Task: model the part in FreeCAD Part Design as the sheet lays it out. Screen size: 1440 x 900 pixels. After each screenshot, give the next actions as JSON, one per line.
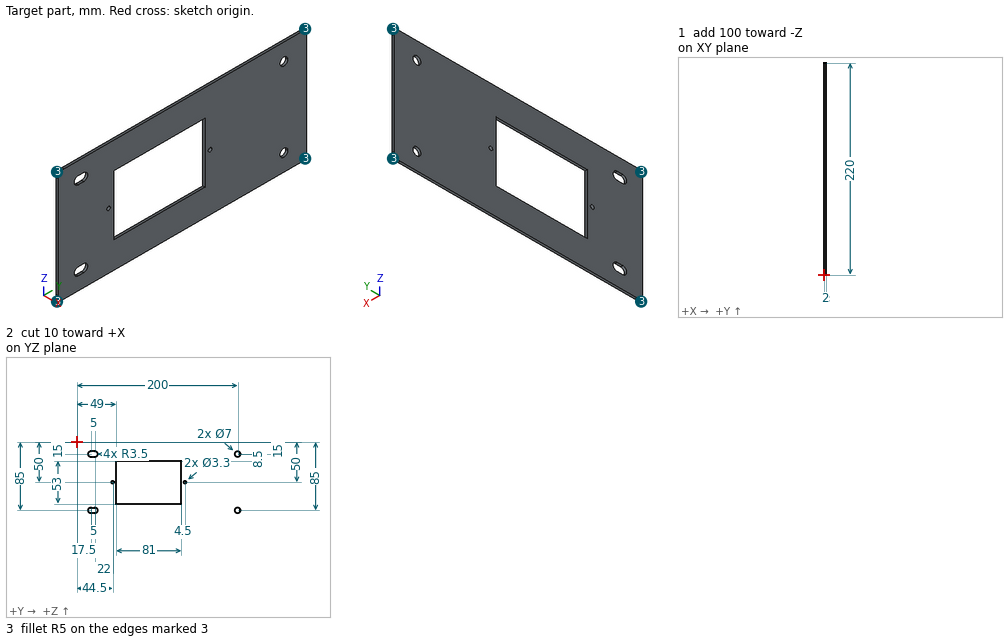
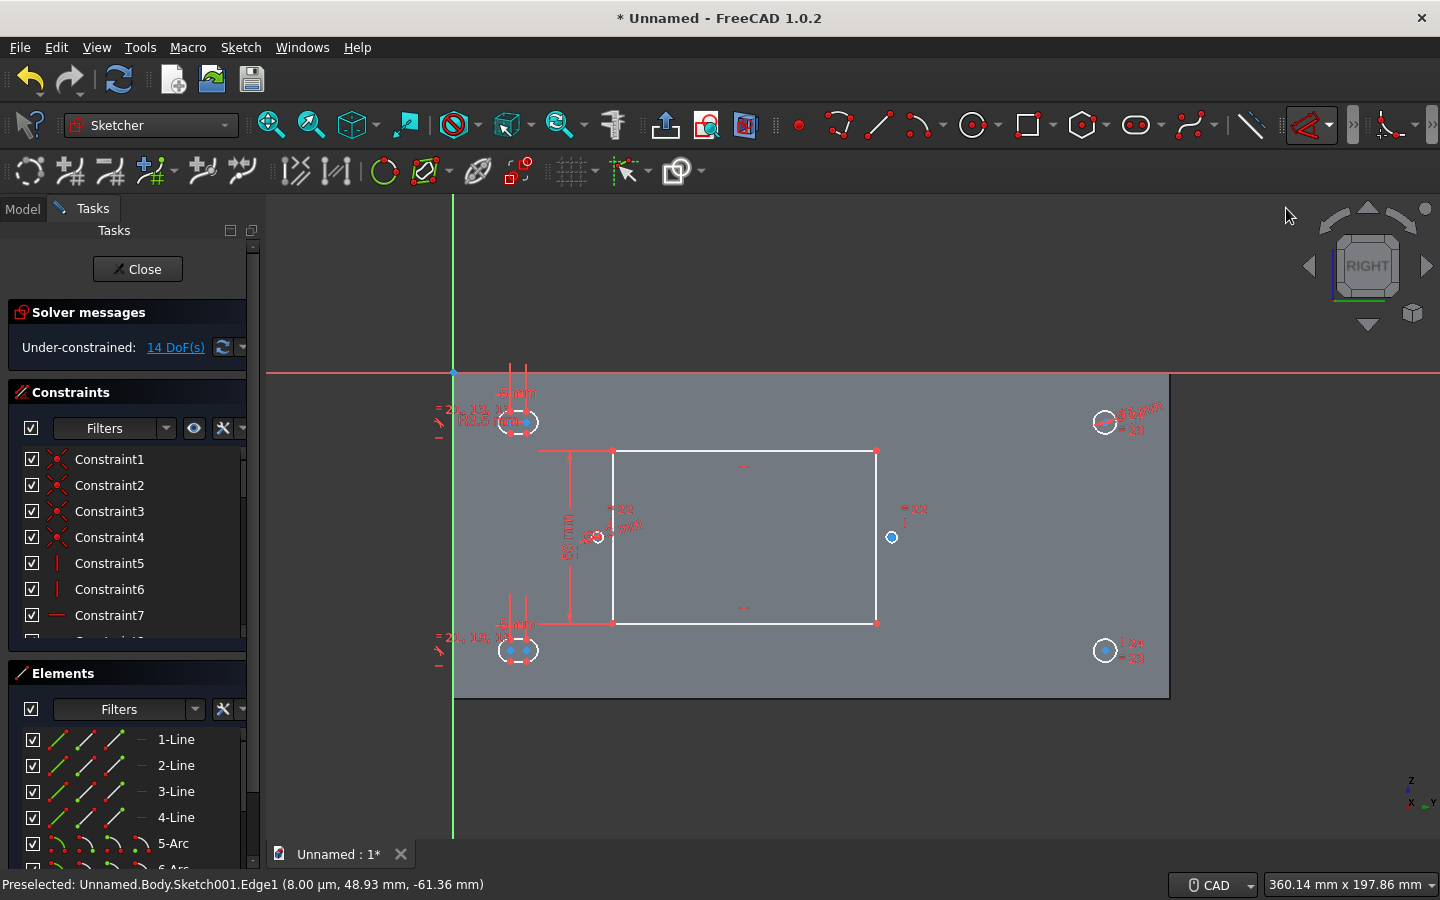
{"action": "left_click", "coordinate": [692, 624]}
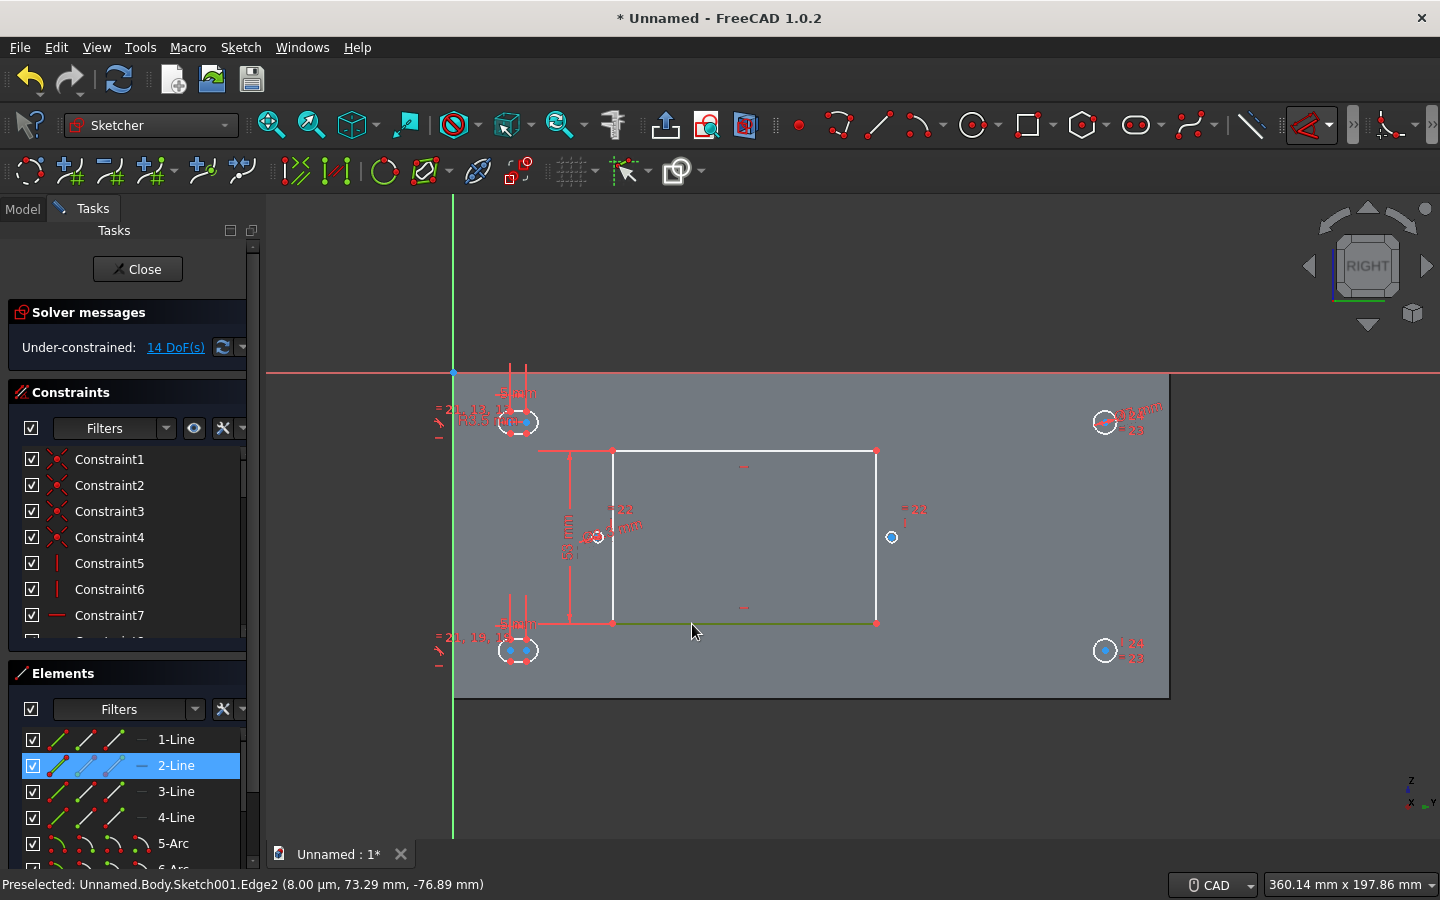
{"action": "left_click", "coordinate": [1332, 126]}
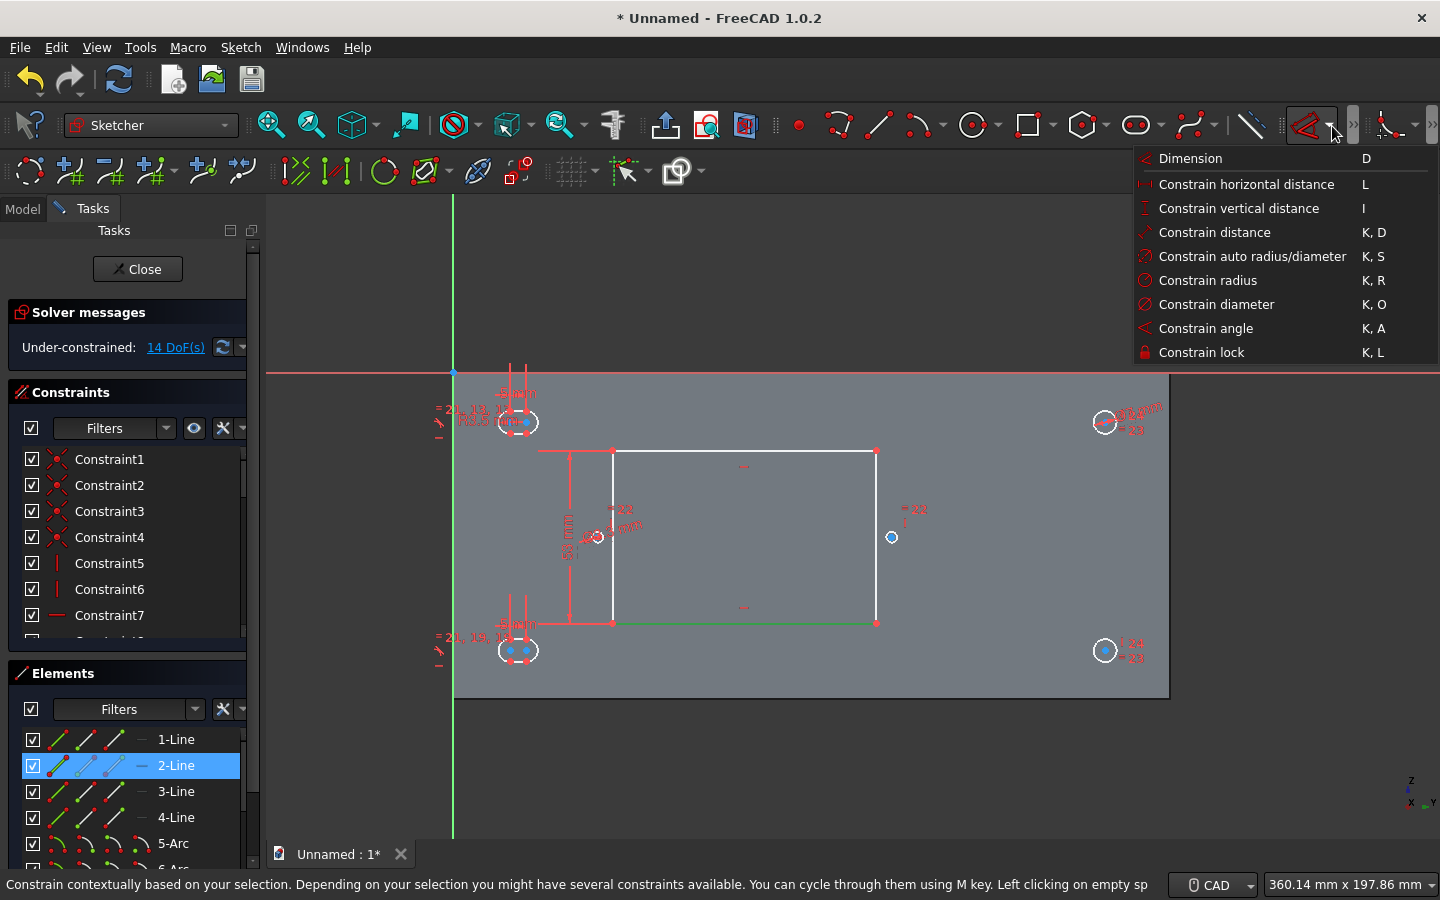
{"action": "left_click", "coordinate": [1286, 184]}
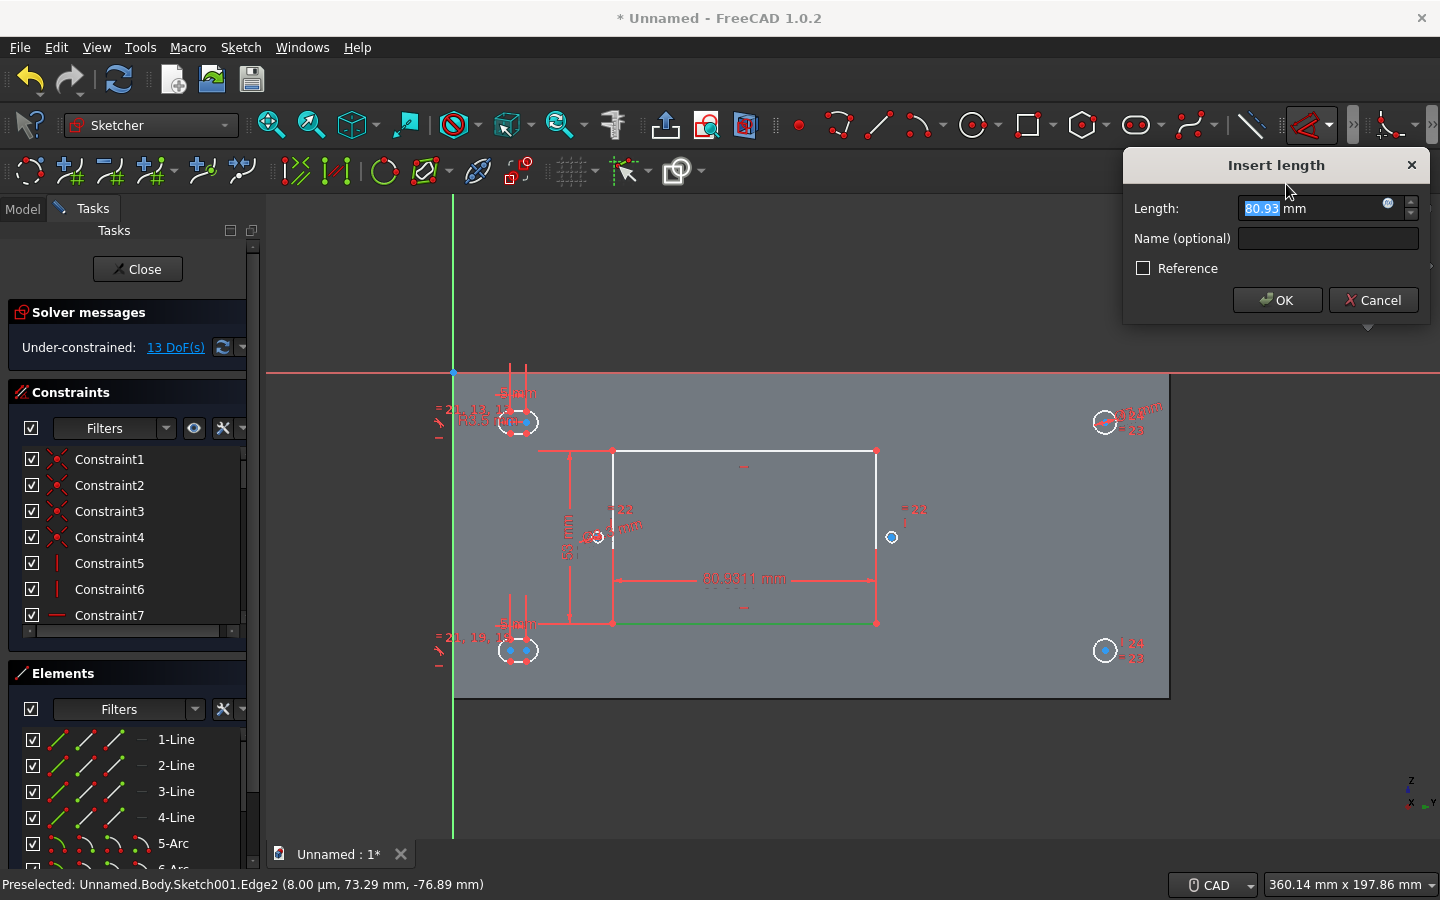
{"action": "type", "text": "81"}
{"action": "key", "text": "Return"}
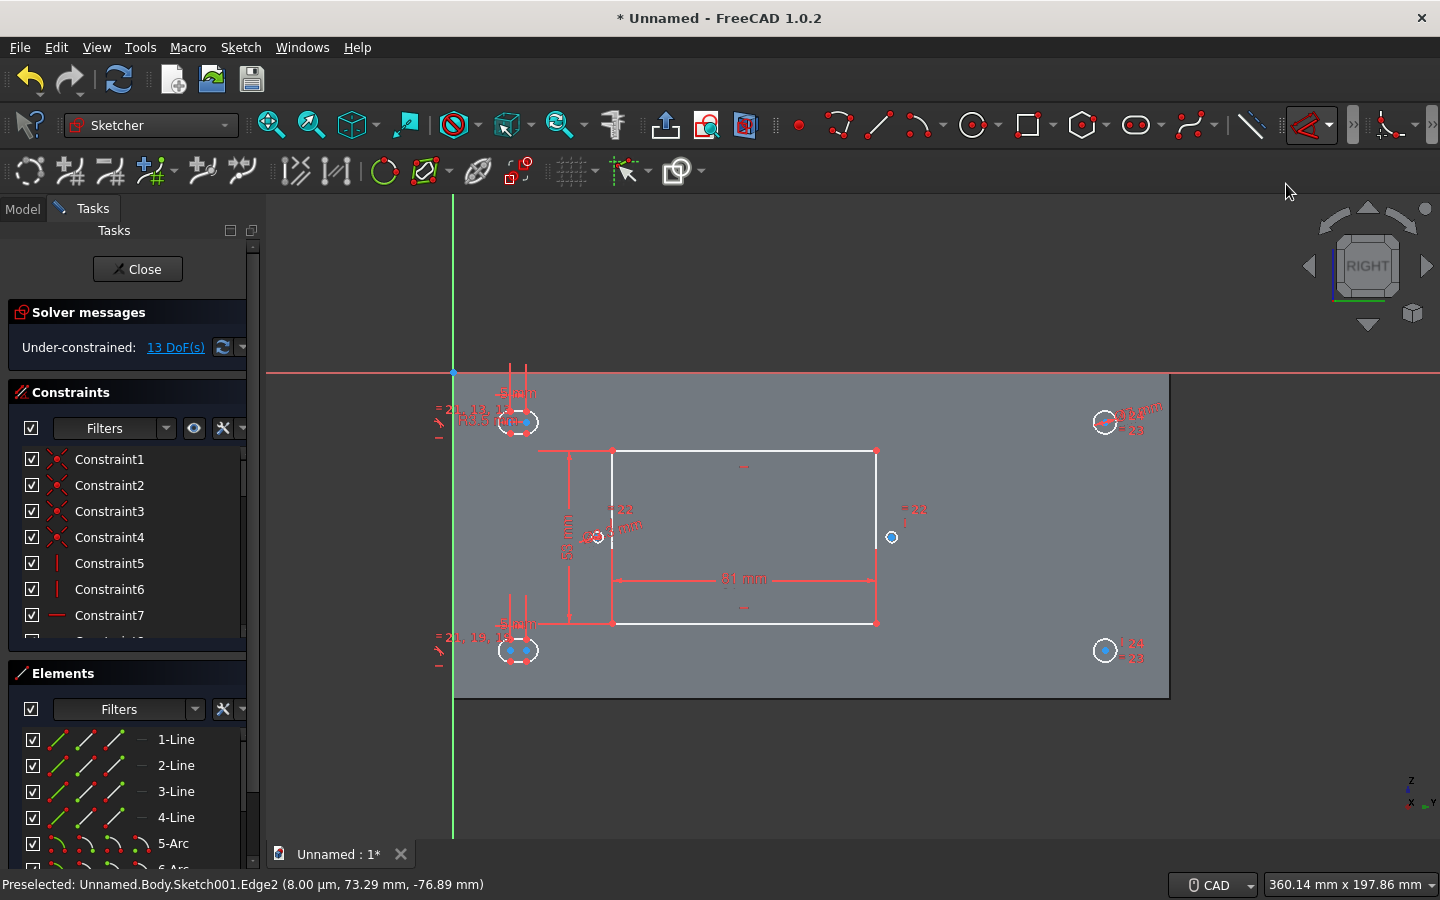
{"action": "left_click", "coordinate": [598, 537]}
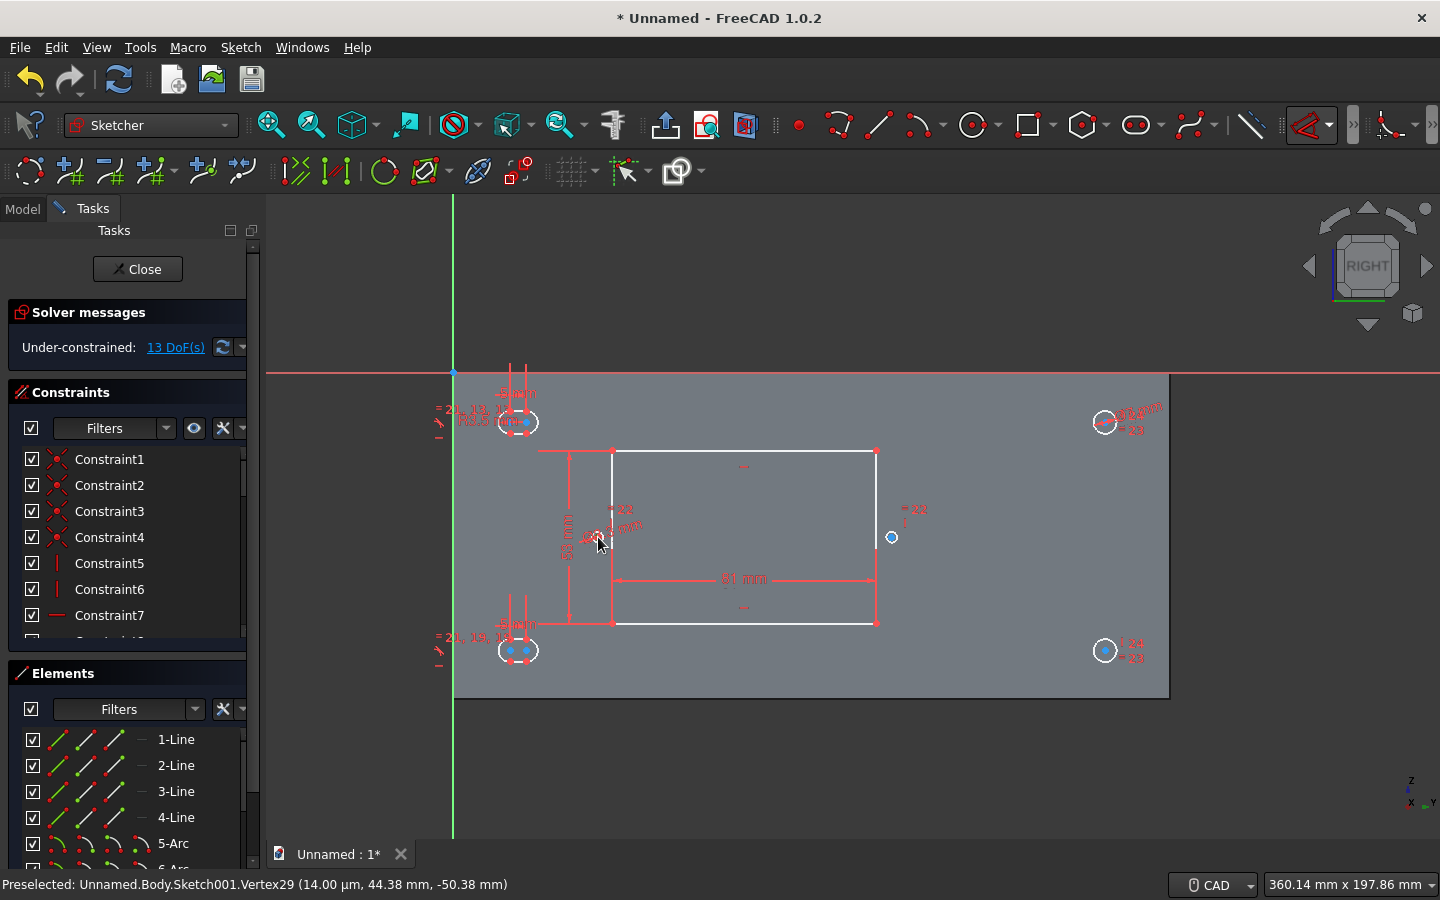
{"action": "left_click", "coordinate": [1332, 126]}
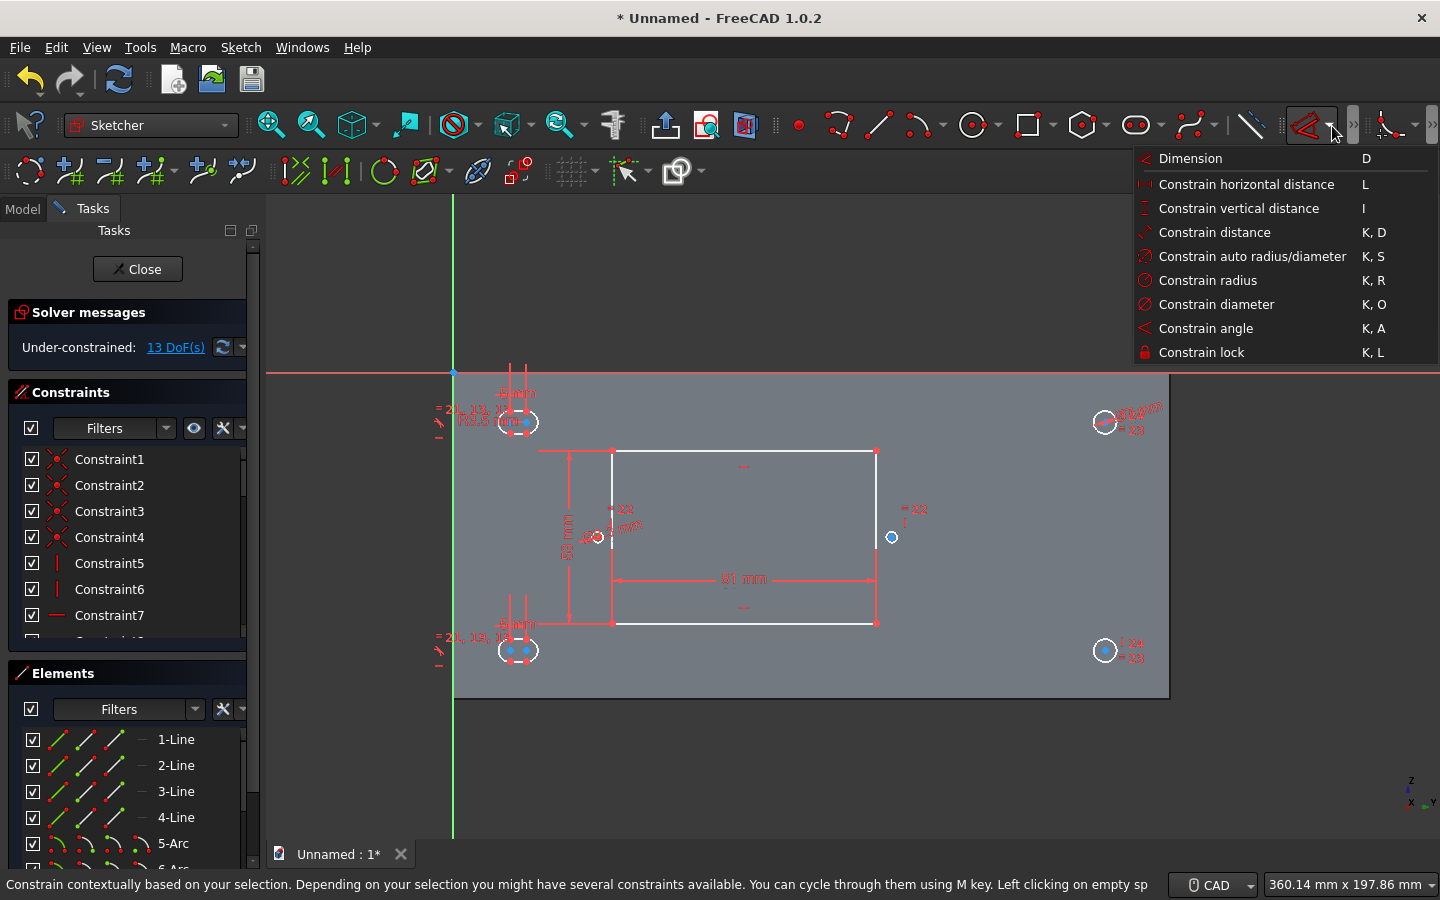
{"action": "left_click", "coordinate": [1286, 208]}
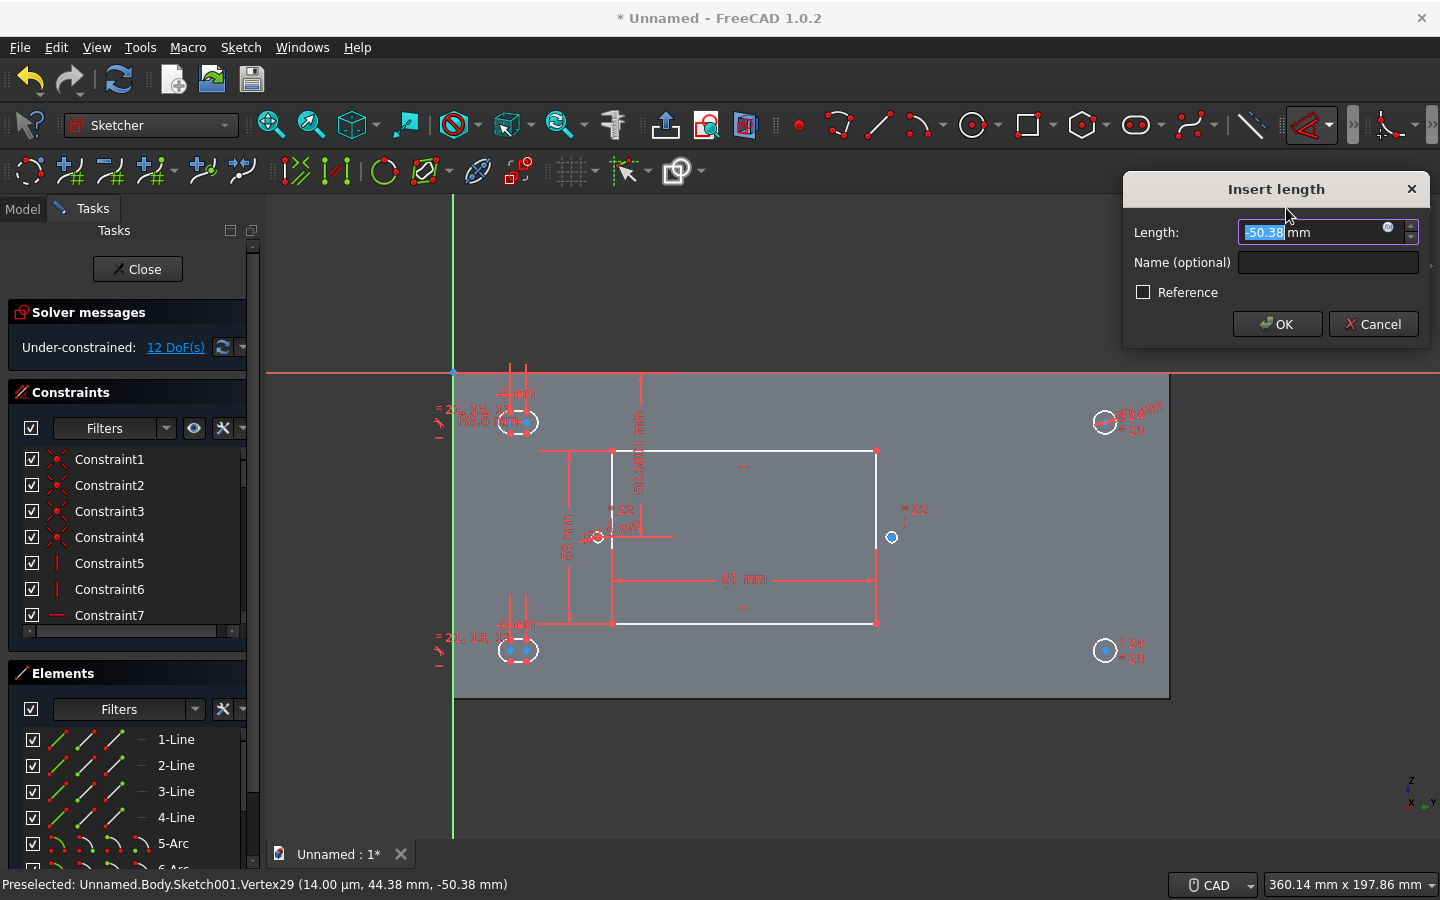
{"action": "type", "text": "-50"}
{"action": "key", "text": "Return"}